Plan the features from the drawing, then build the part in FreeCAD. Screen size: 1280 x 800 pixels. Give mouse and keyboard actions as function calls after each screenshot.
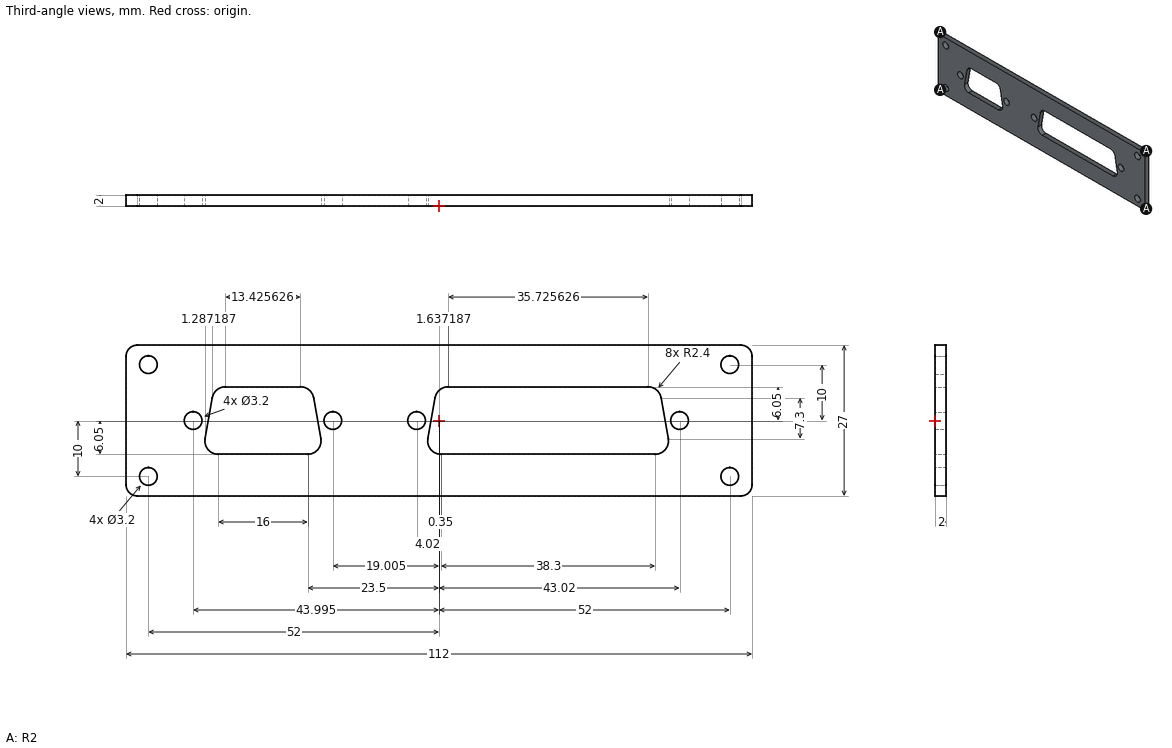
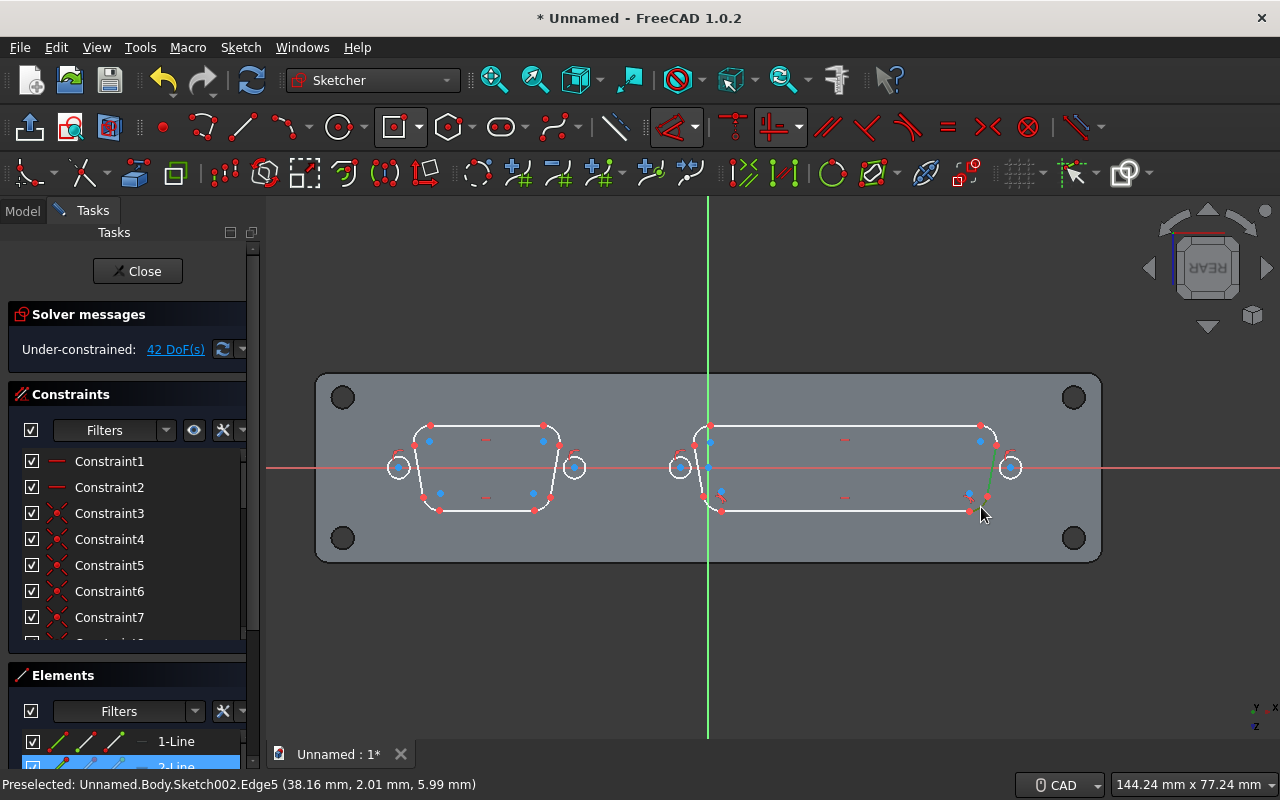
key(t)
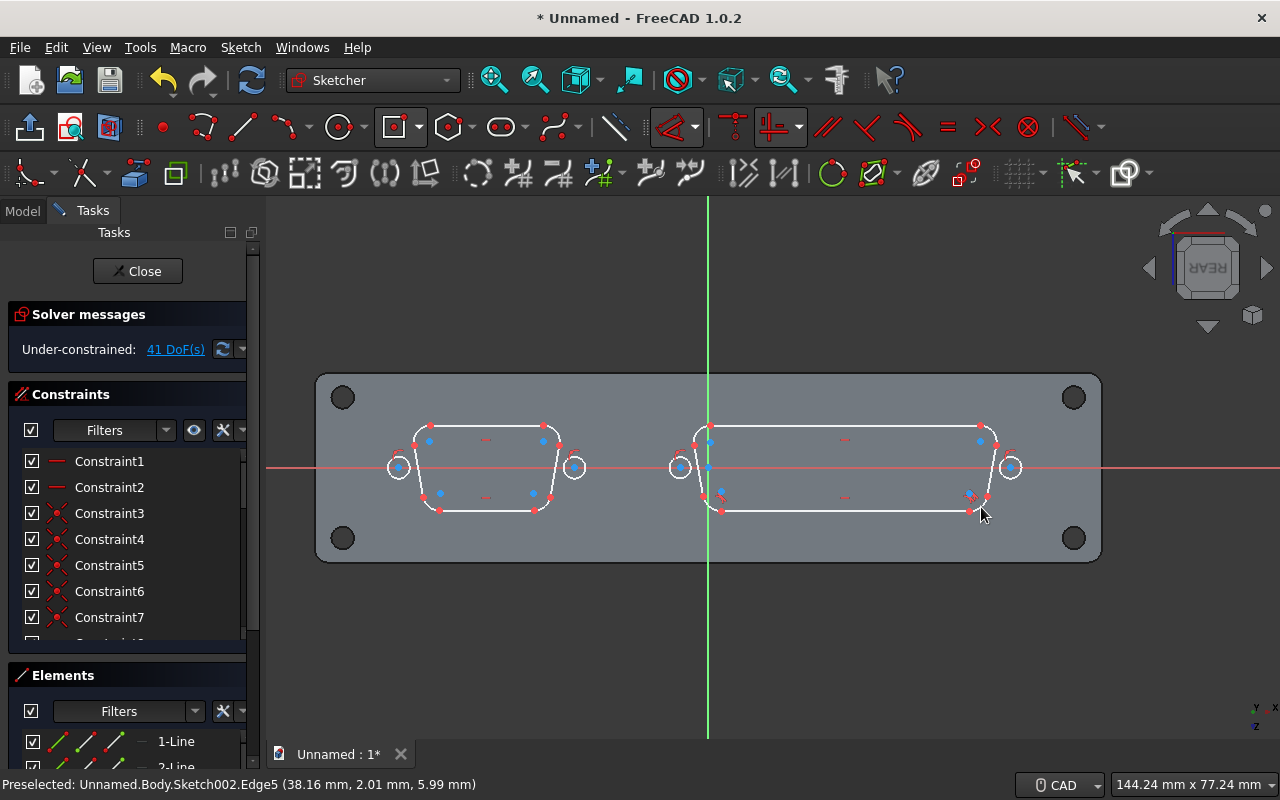
click(990, 481)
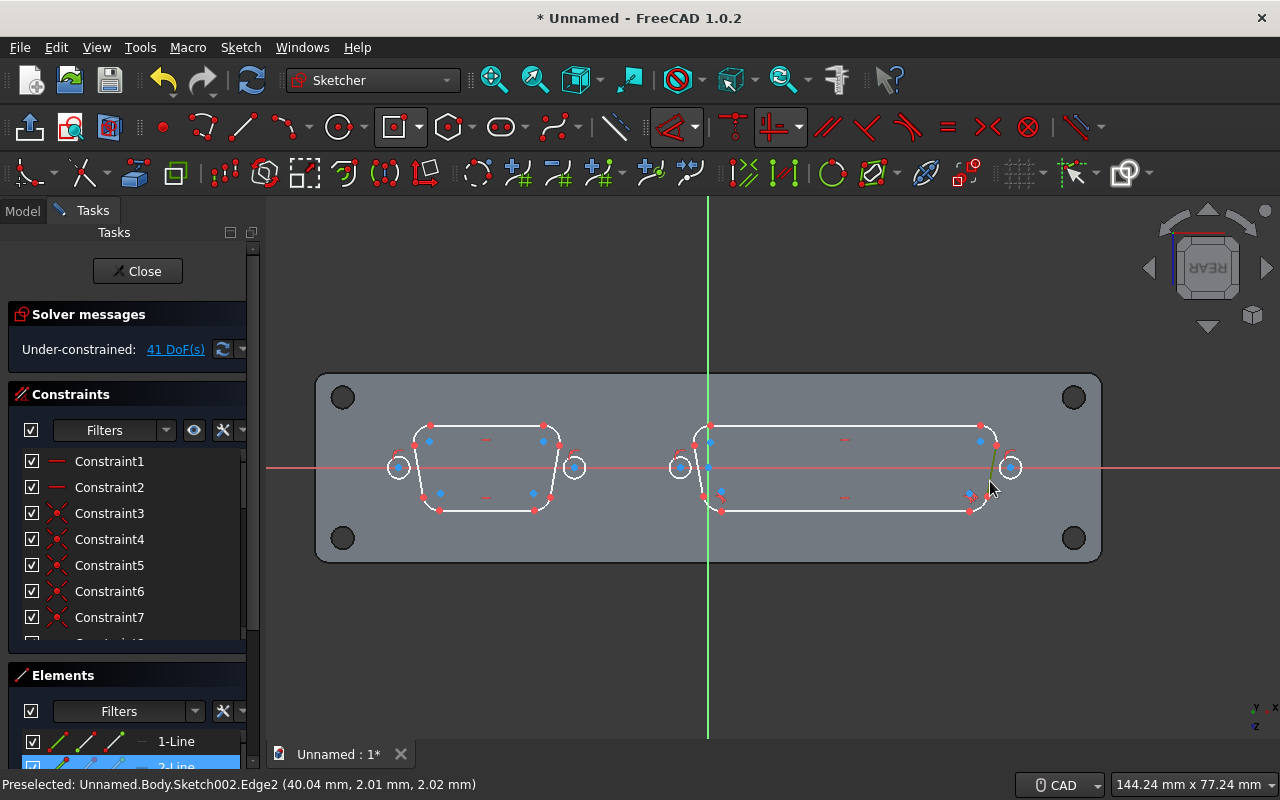
click(993, 432)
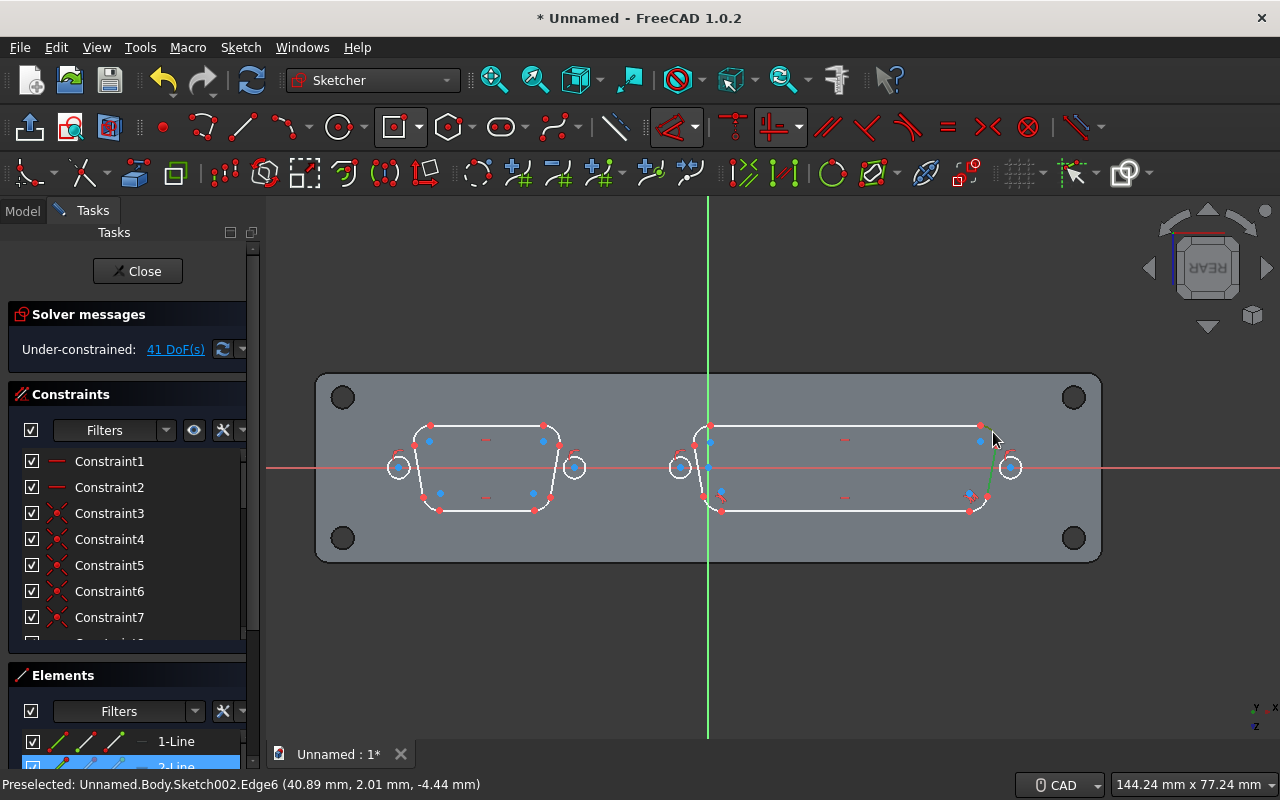
click(908, 128)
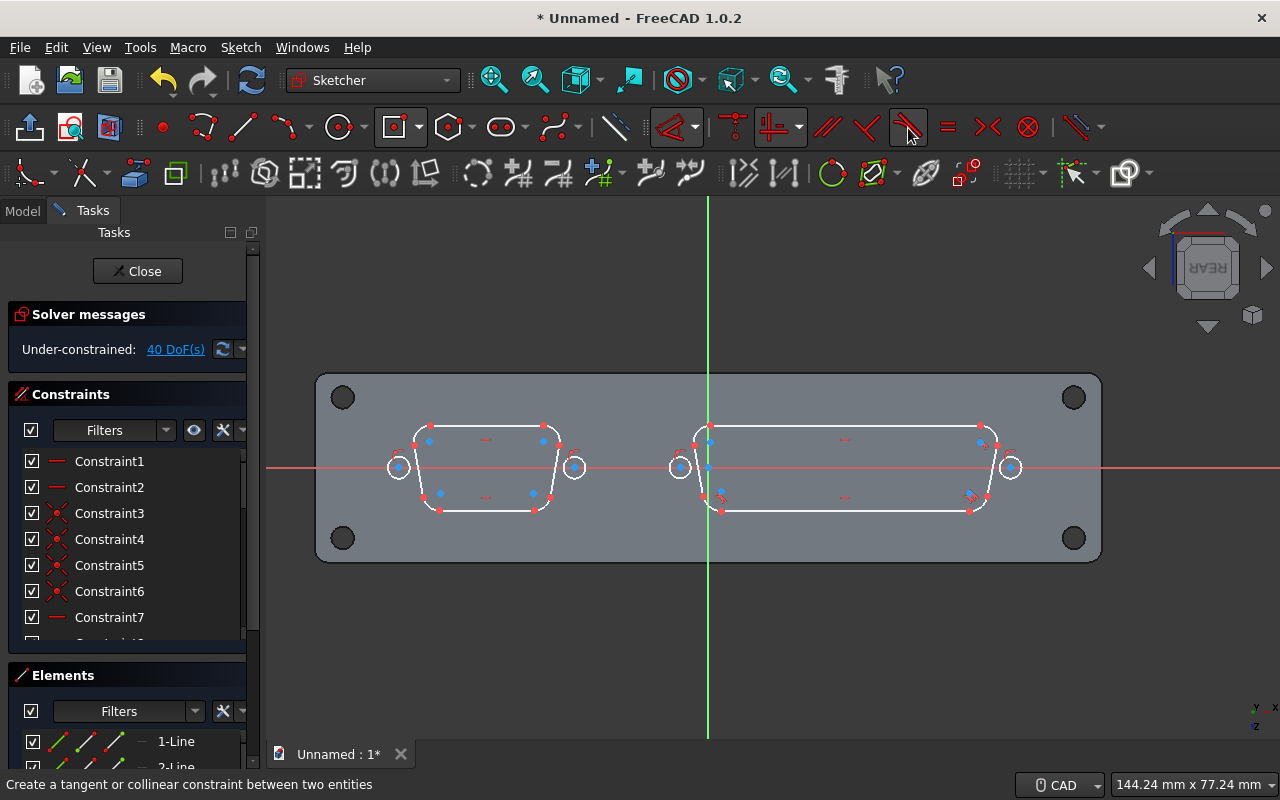
click(899, 426)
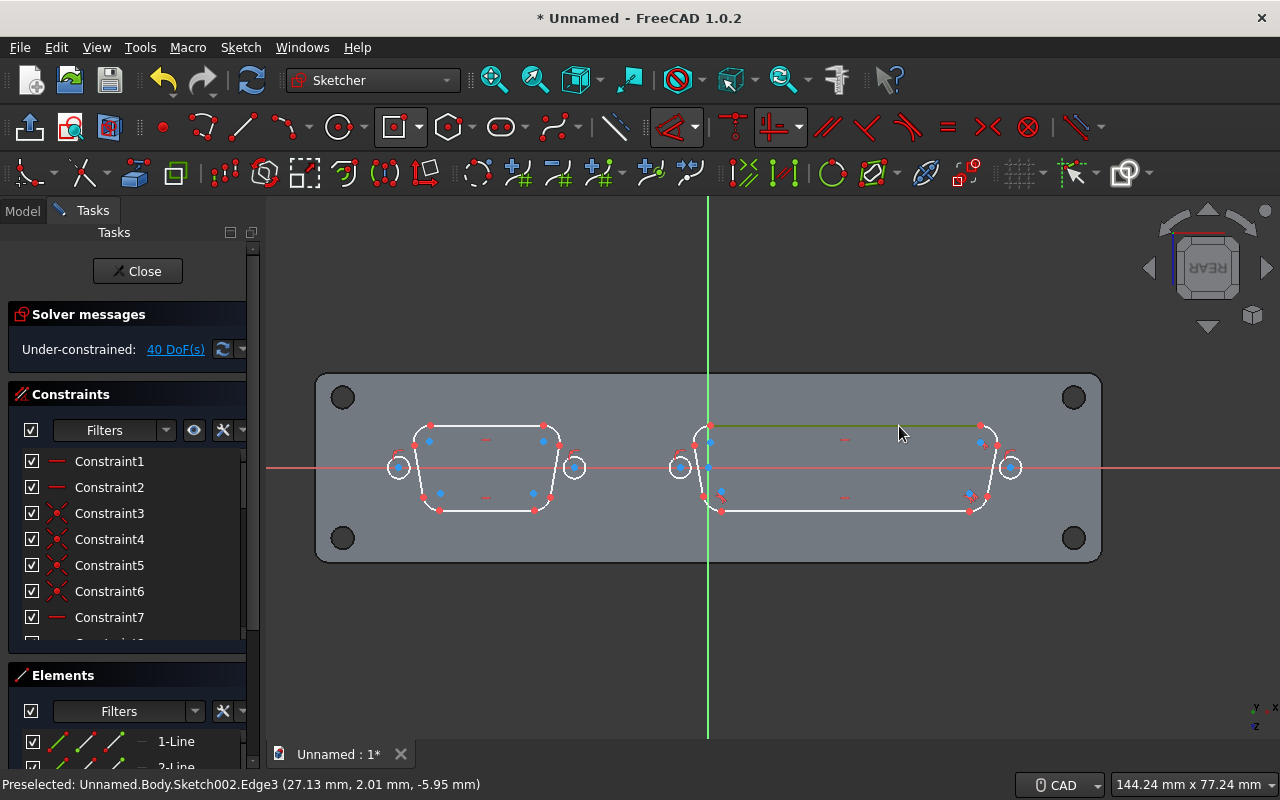
click(993, 432)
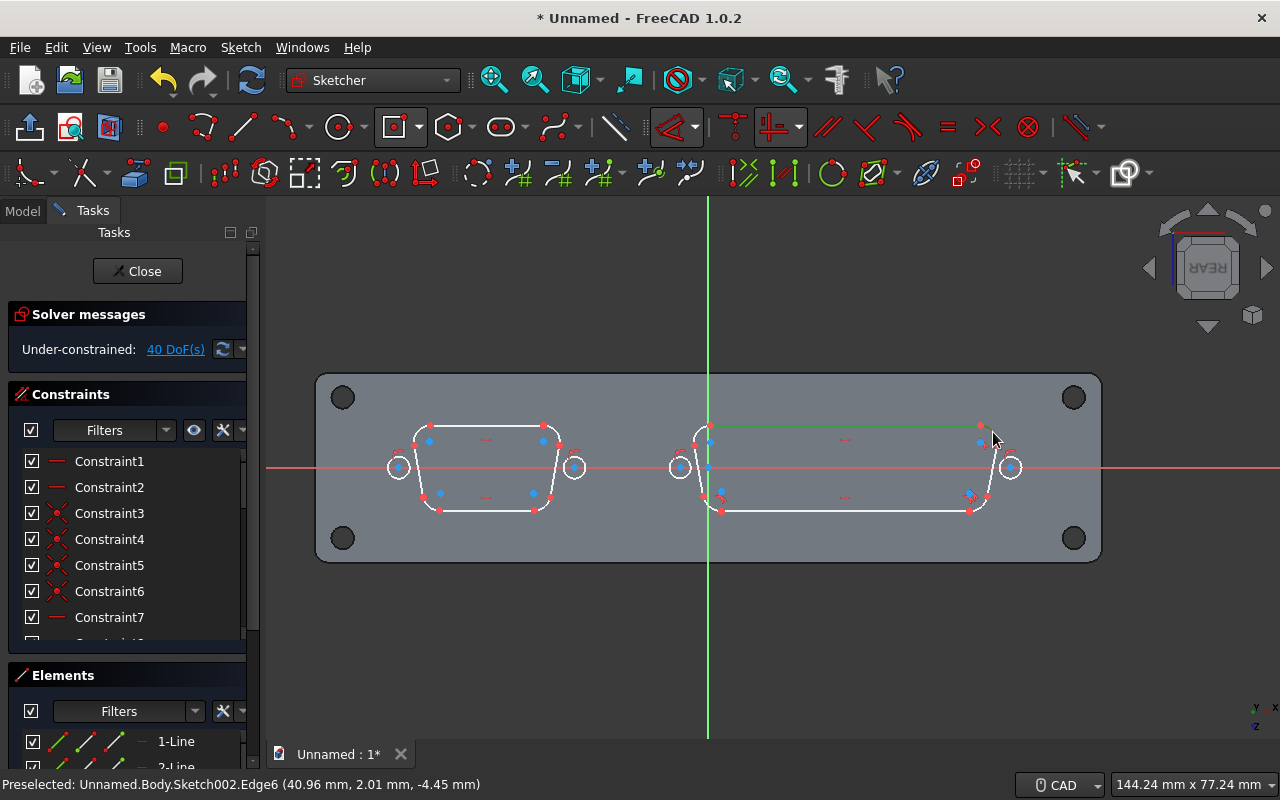
click(908, 128)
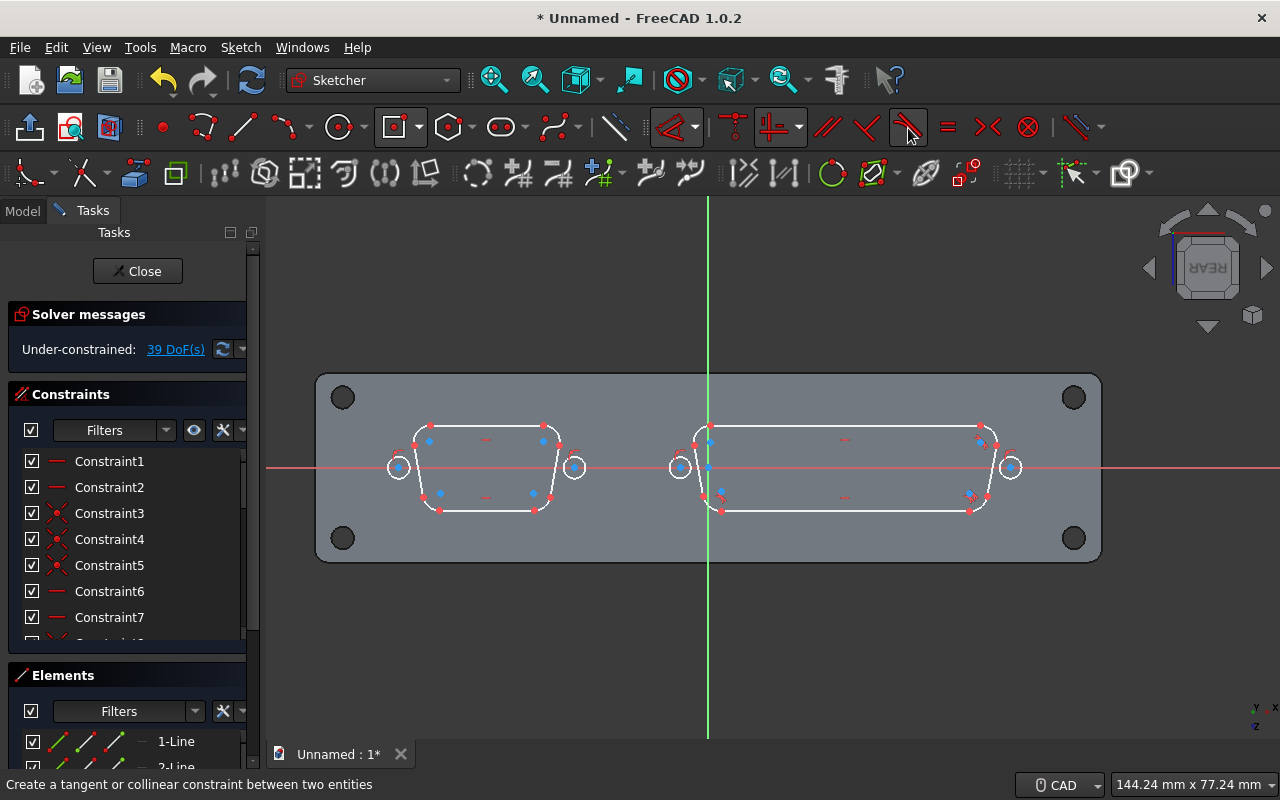
click(899, 426)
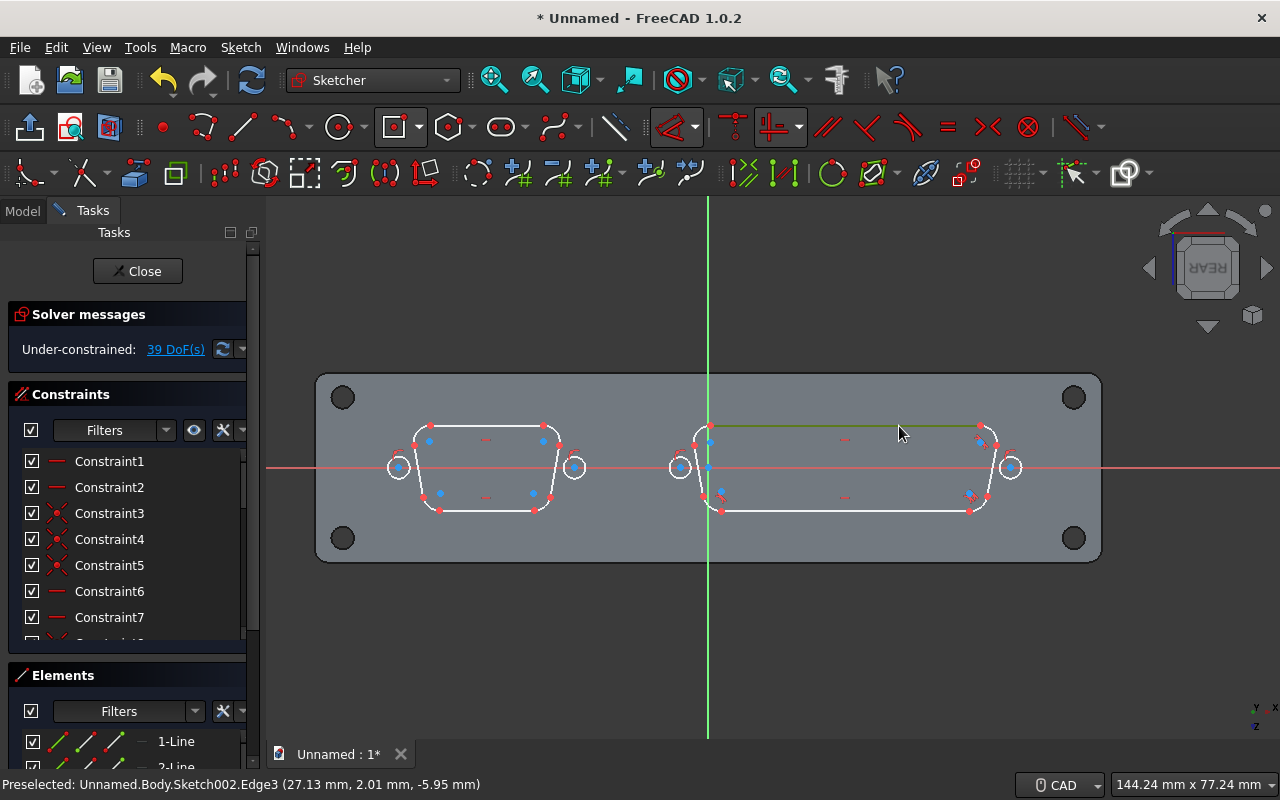
scroll(697, 432, up, 2)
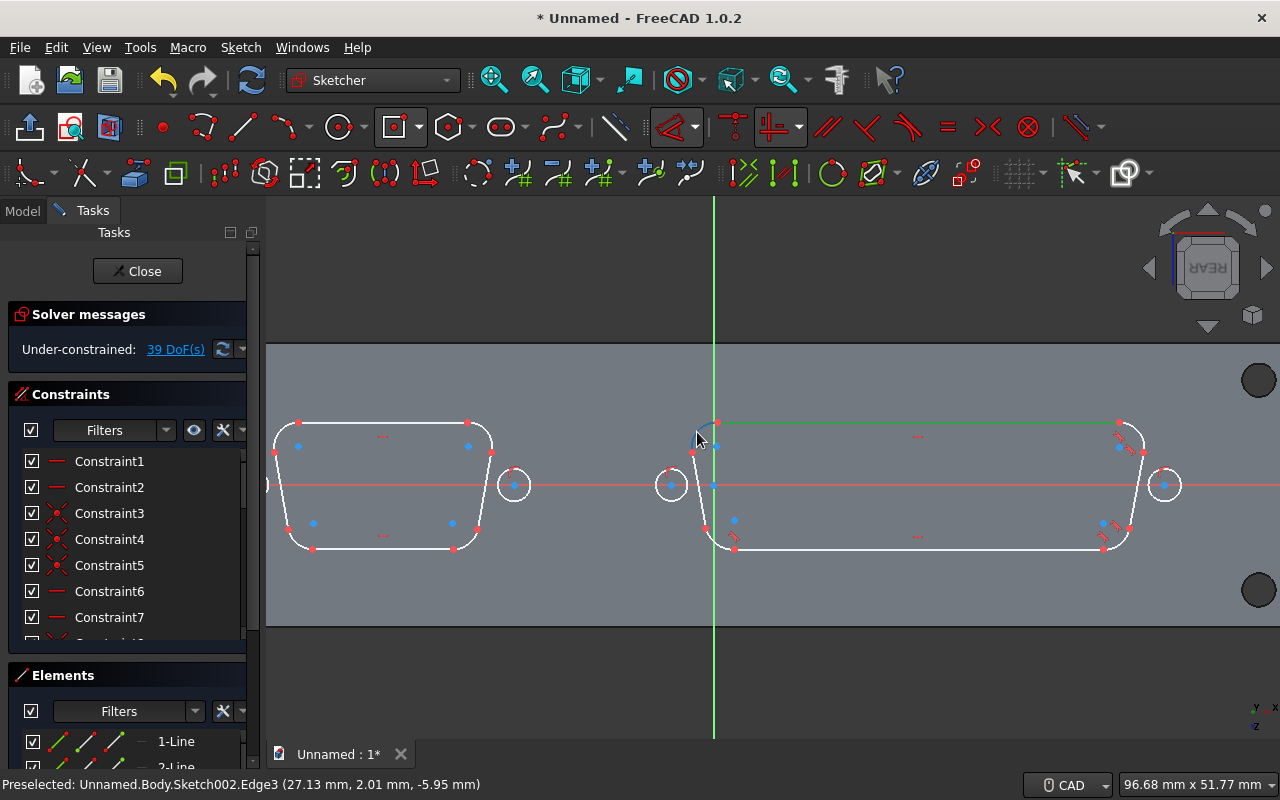
click(697, 431)